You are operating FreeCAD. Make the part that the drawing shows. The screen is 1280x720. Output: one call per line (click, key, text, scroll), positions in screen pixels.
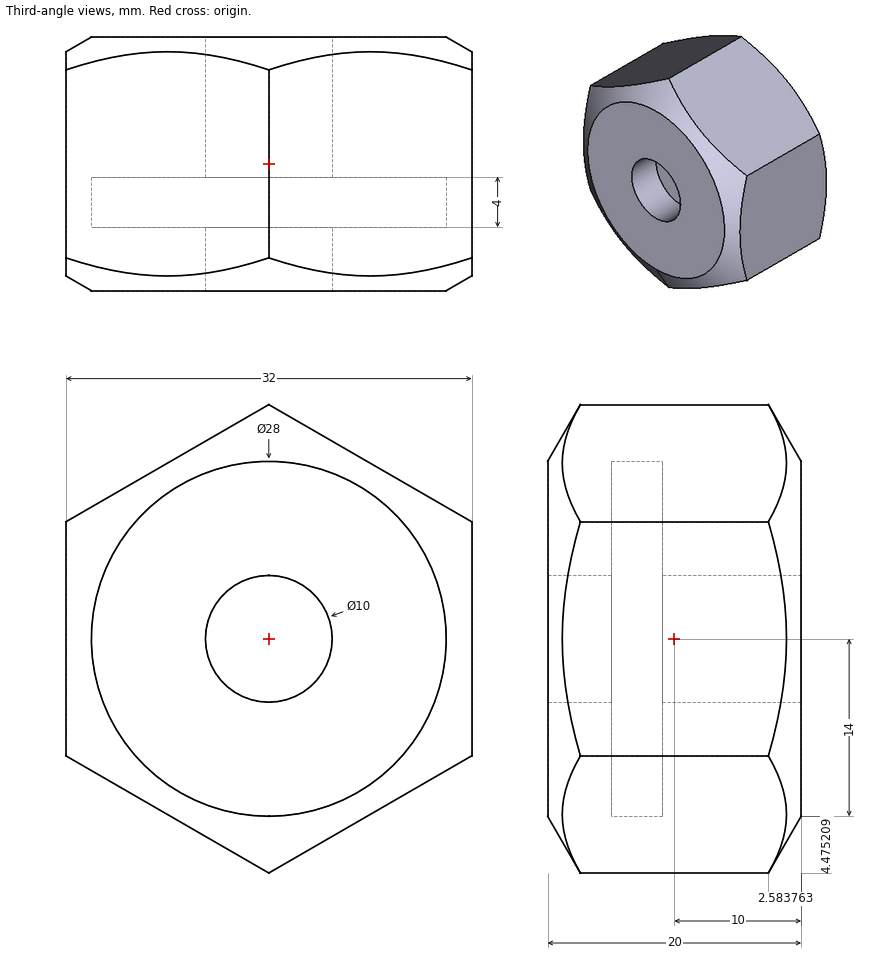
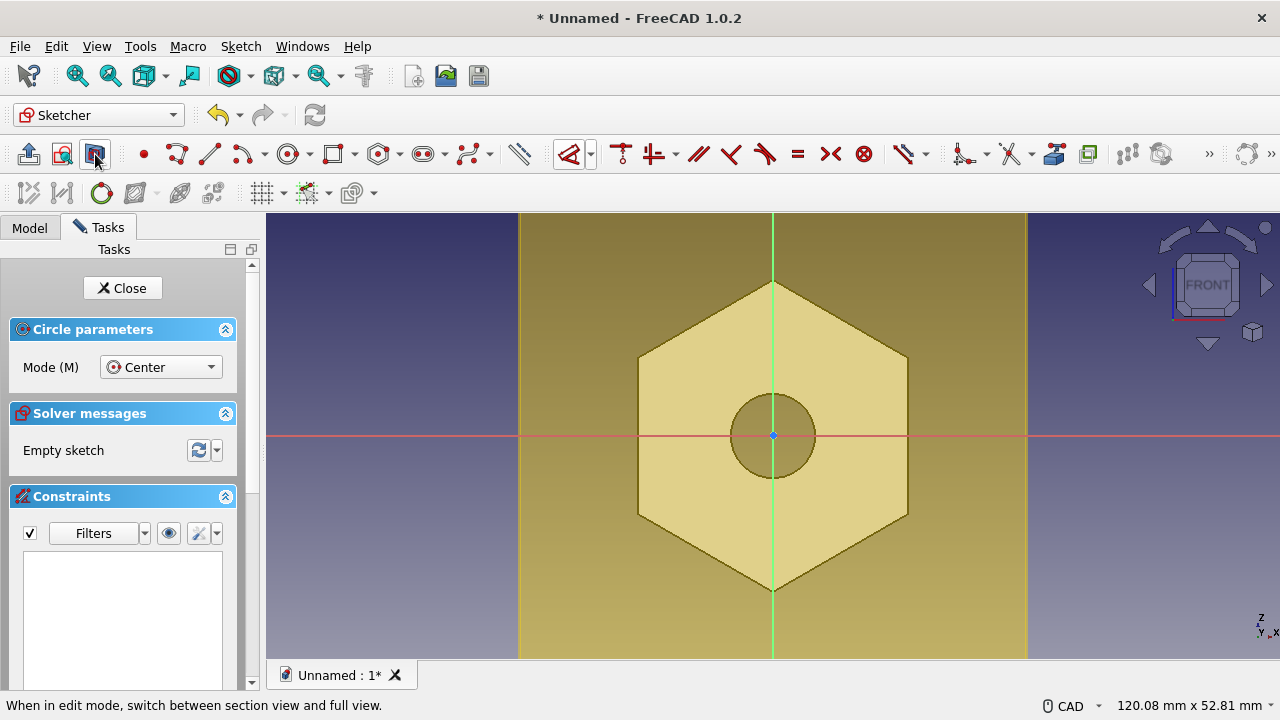
click(773, 436)
click(857, 352)
key(Escape)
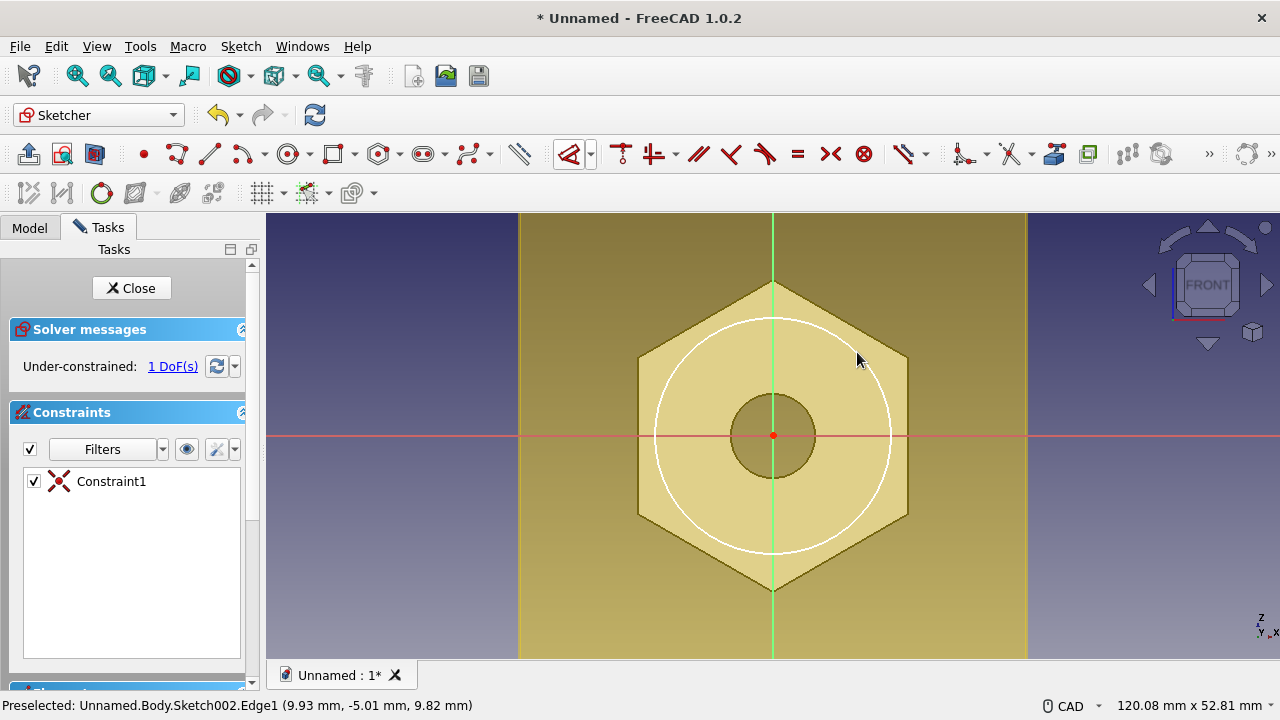
click(856, 352)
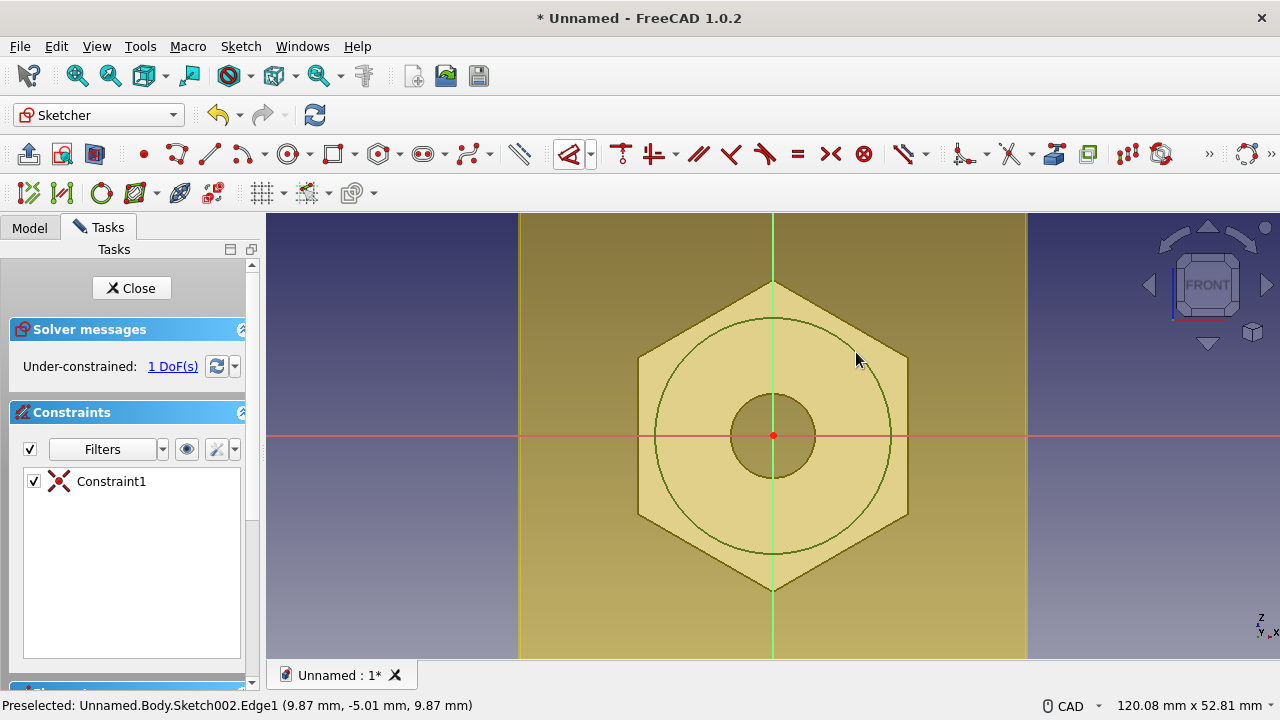
key(k)
key(o)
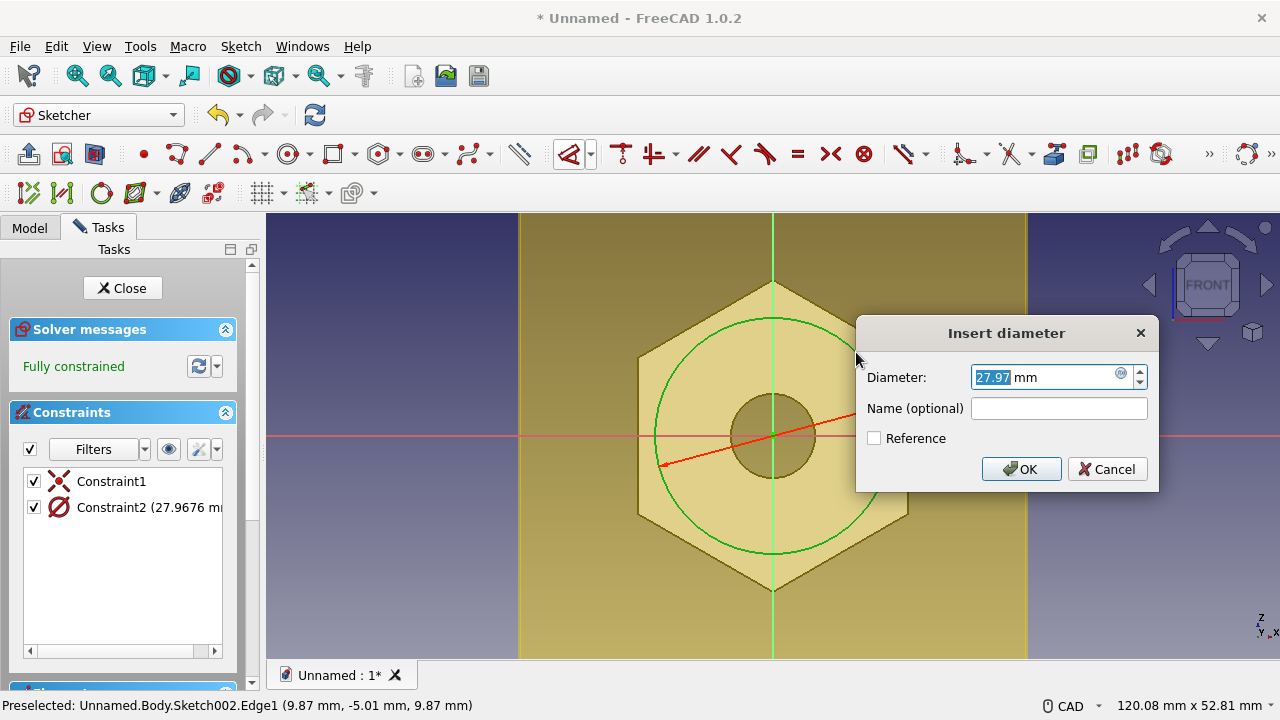
text(28)
key(Return)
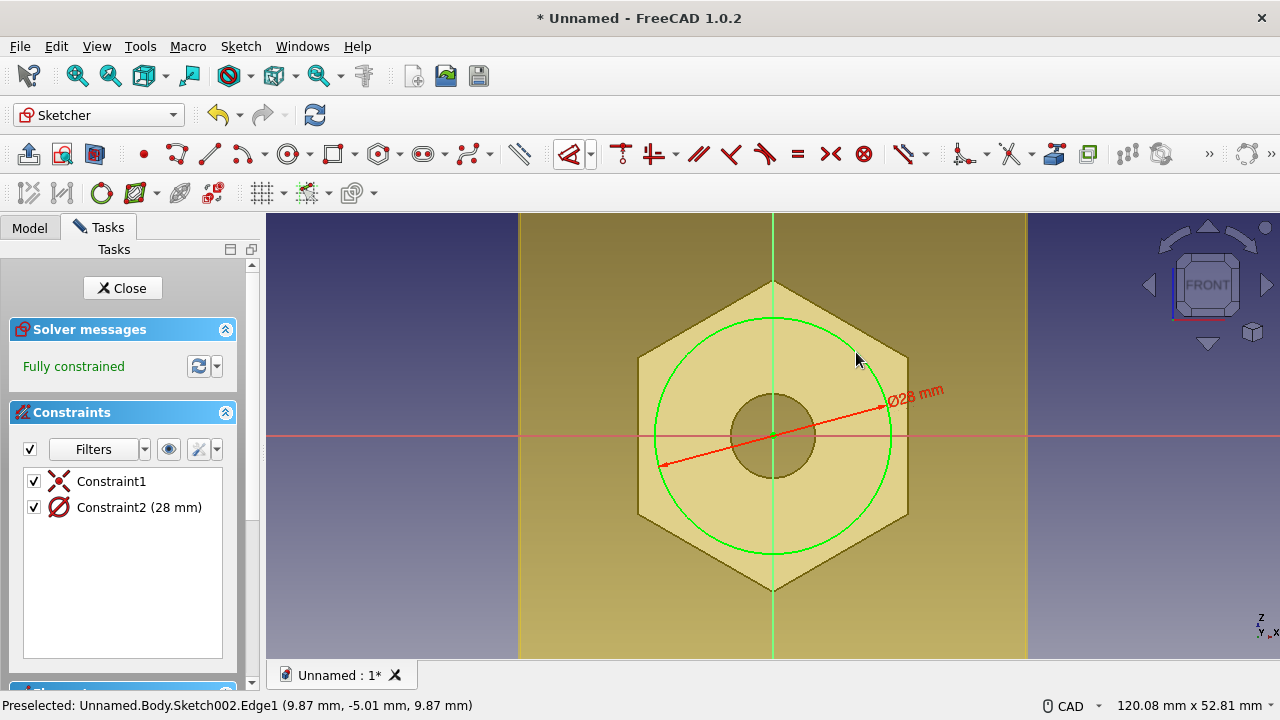
click(123, 288)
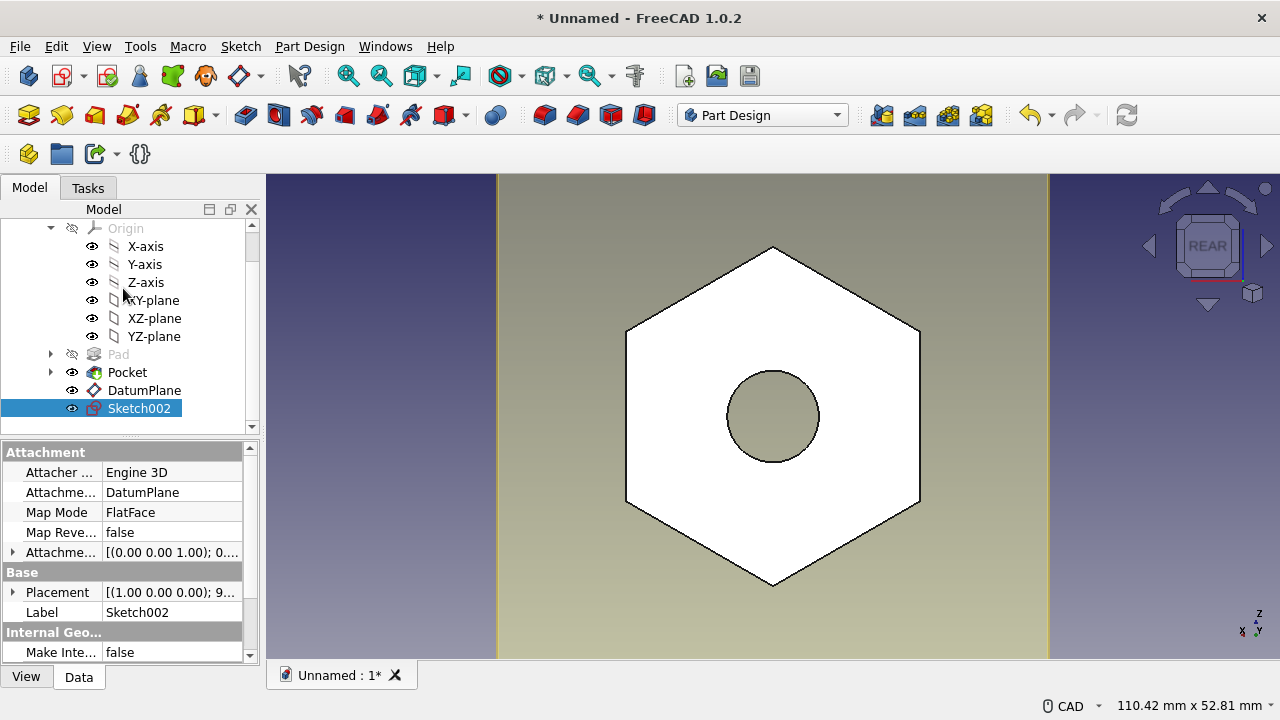
click(246, 116)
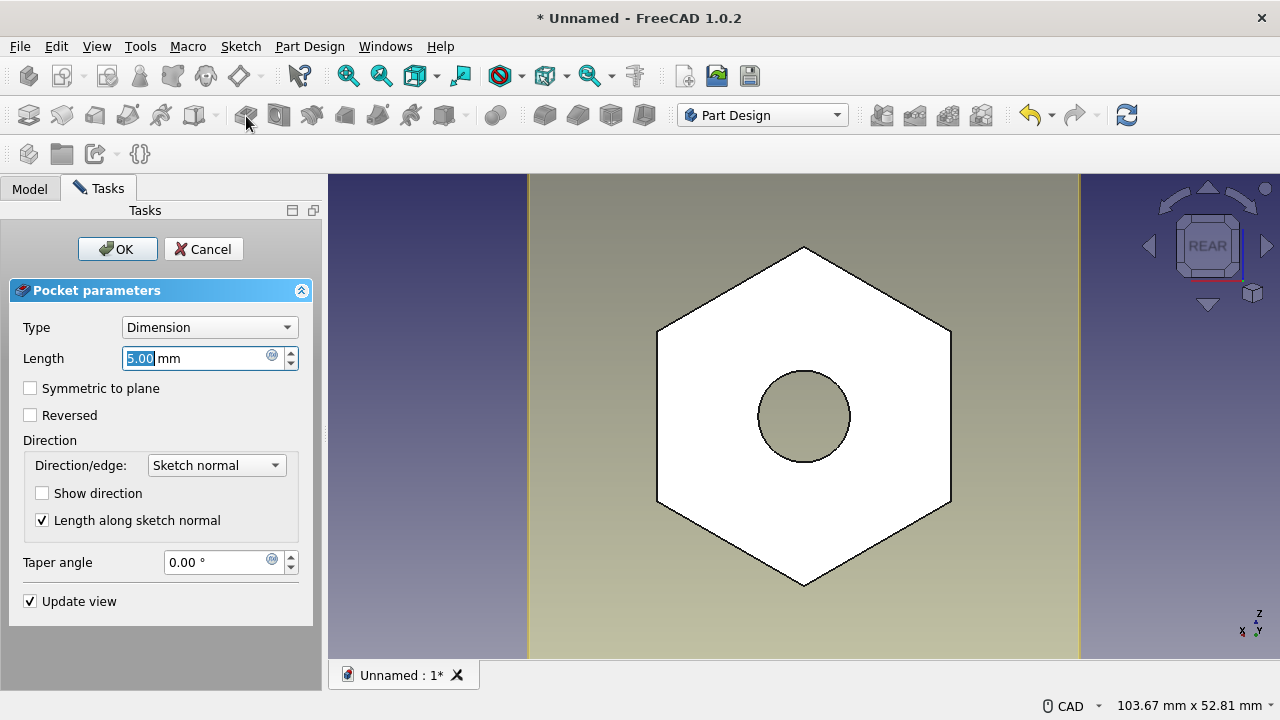
text(4)
key(Tab)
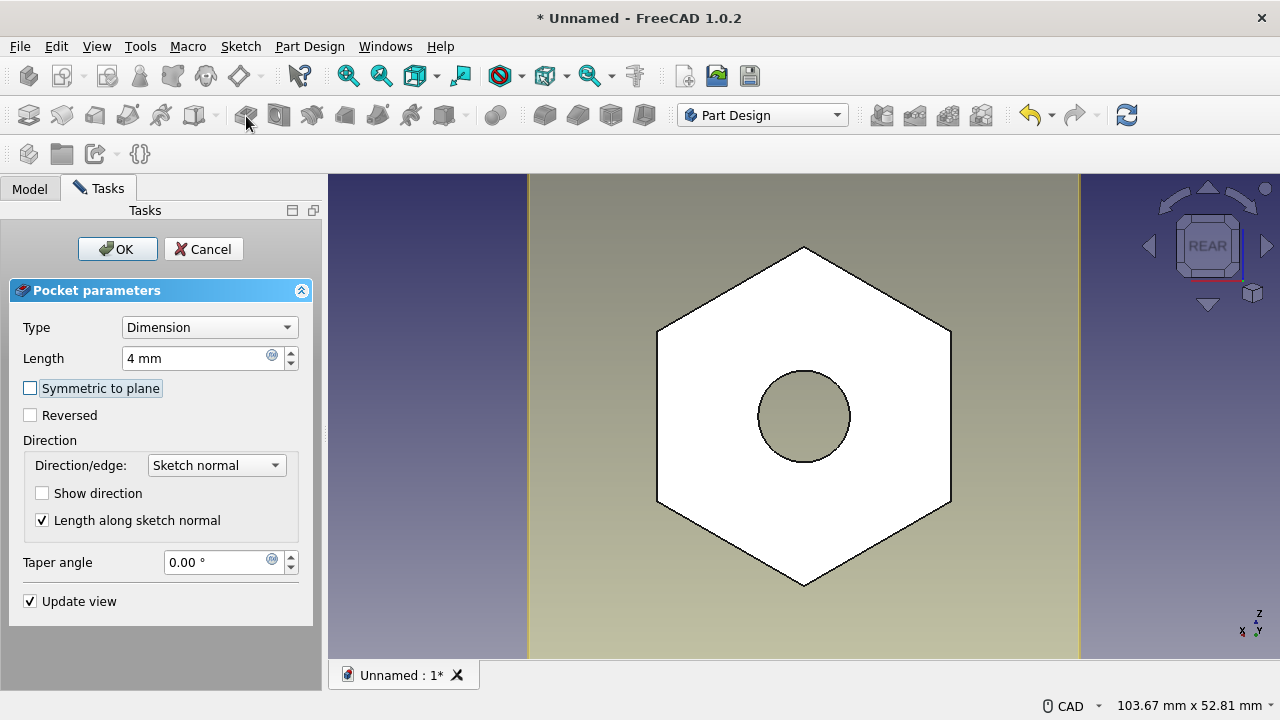
click(118, 249)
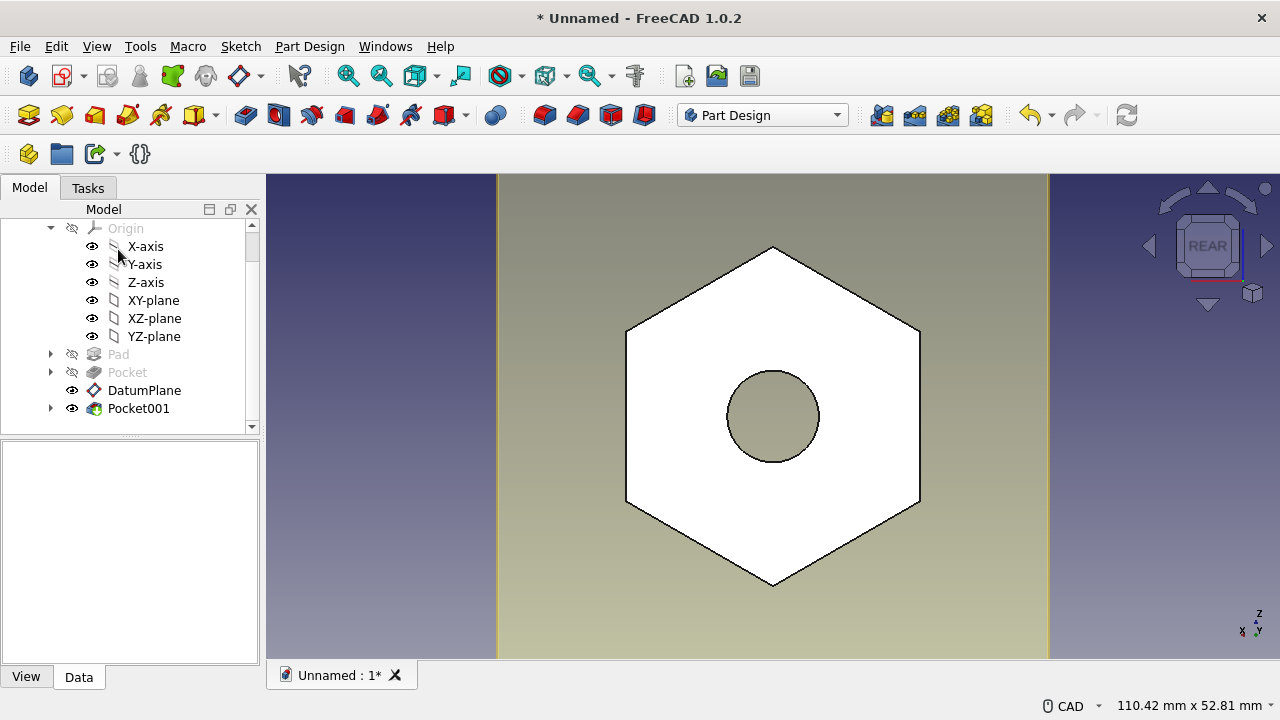
click(117, 390)
key(space)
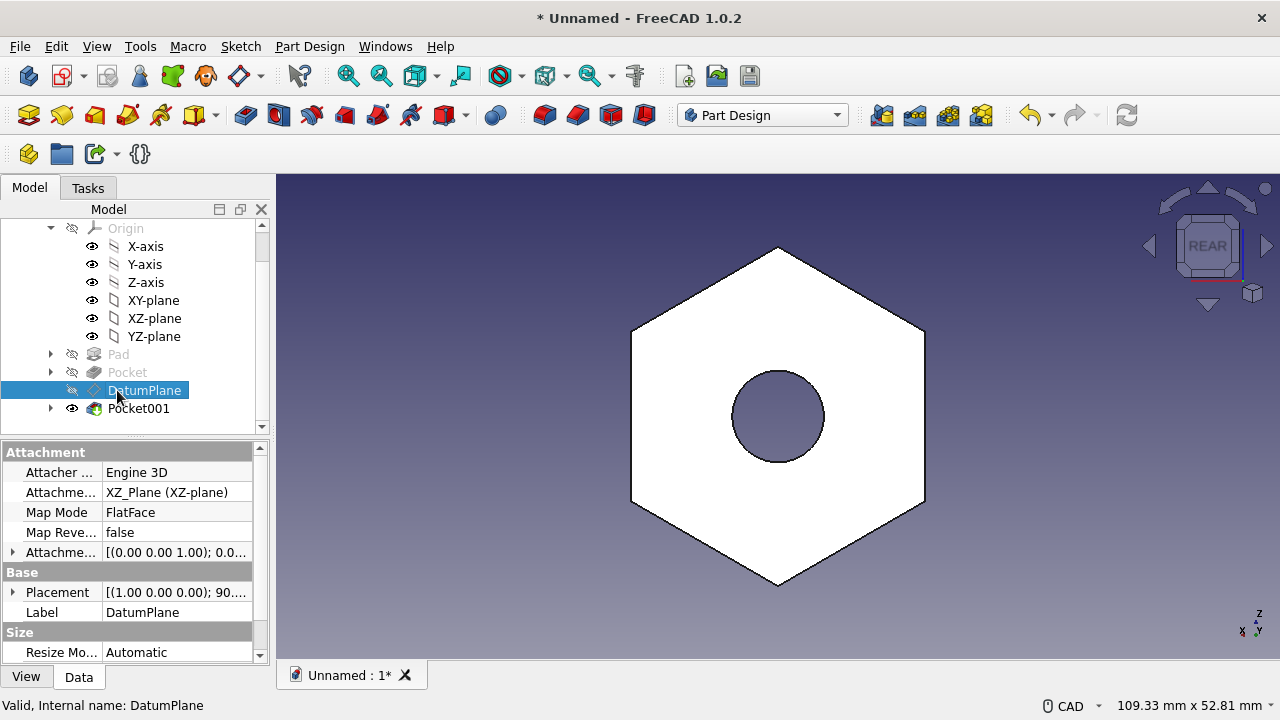
click(316, 619)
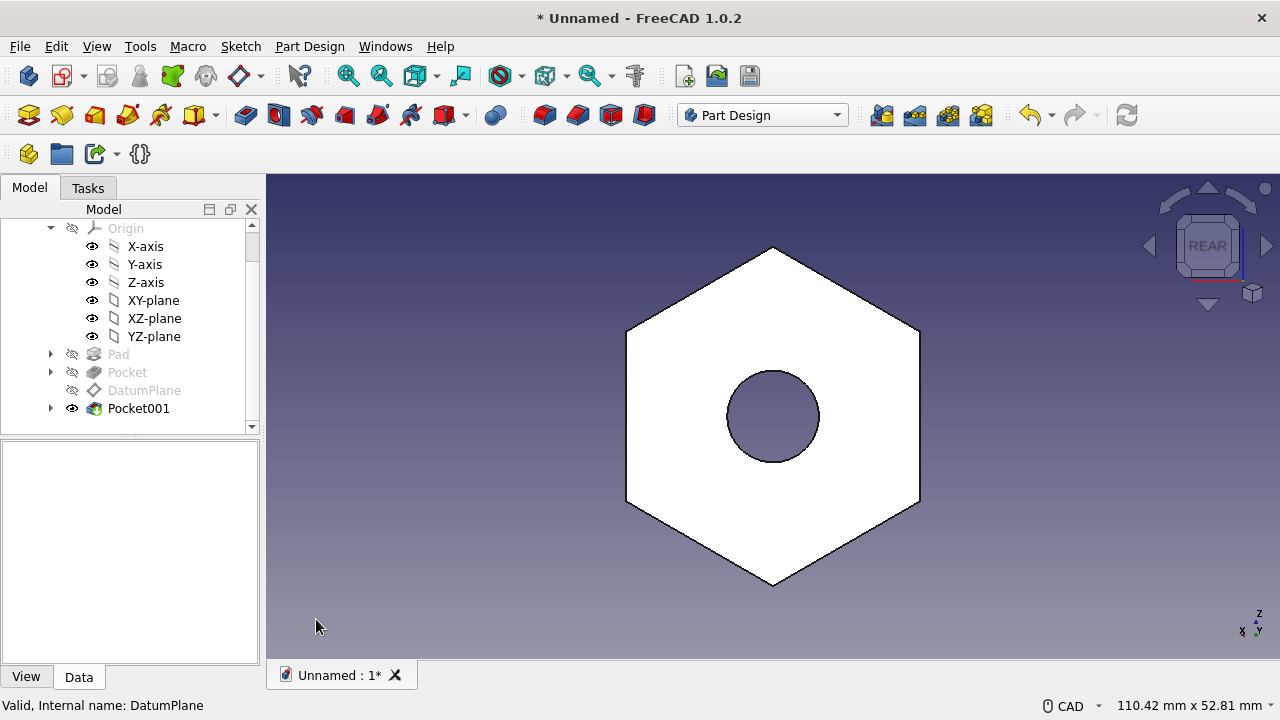
click(62, 76)